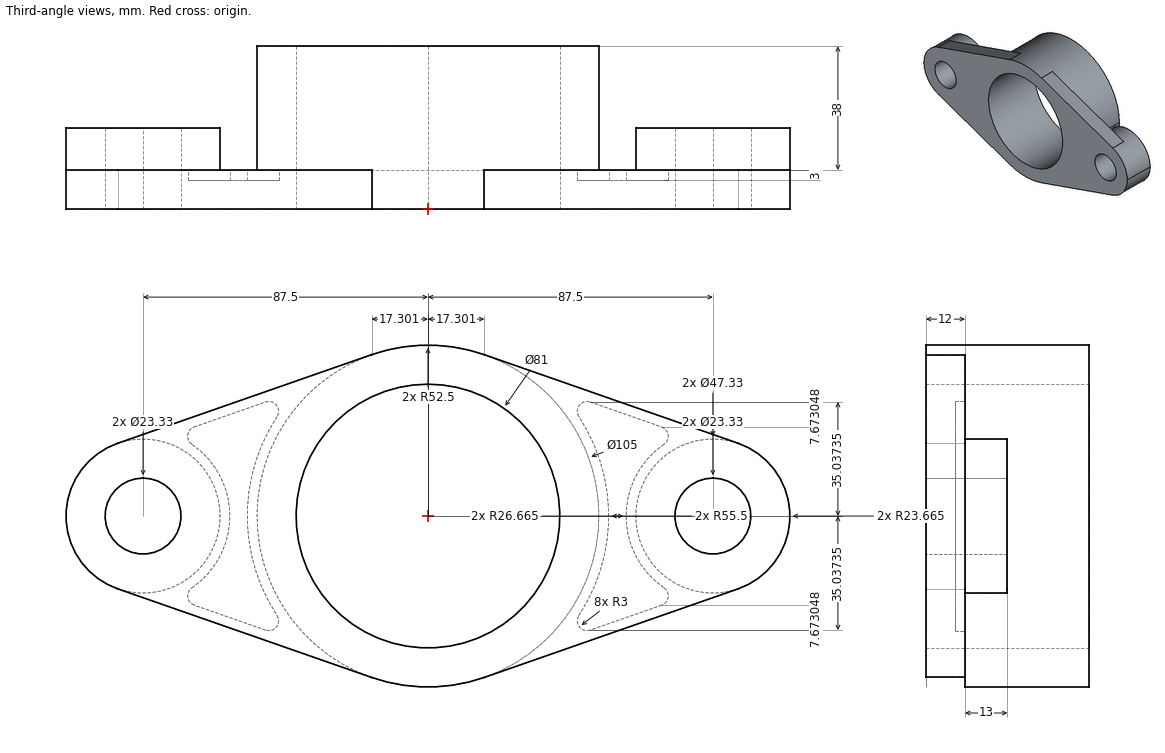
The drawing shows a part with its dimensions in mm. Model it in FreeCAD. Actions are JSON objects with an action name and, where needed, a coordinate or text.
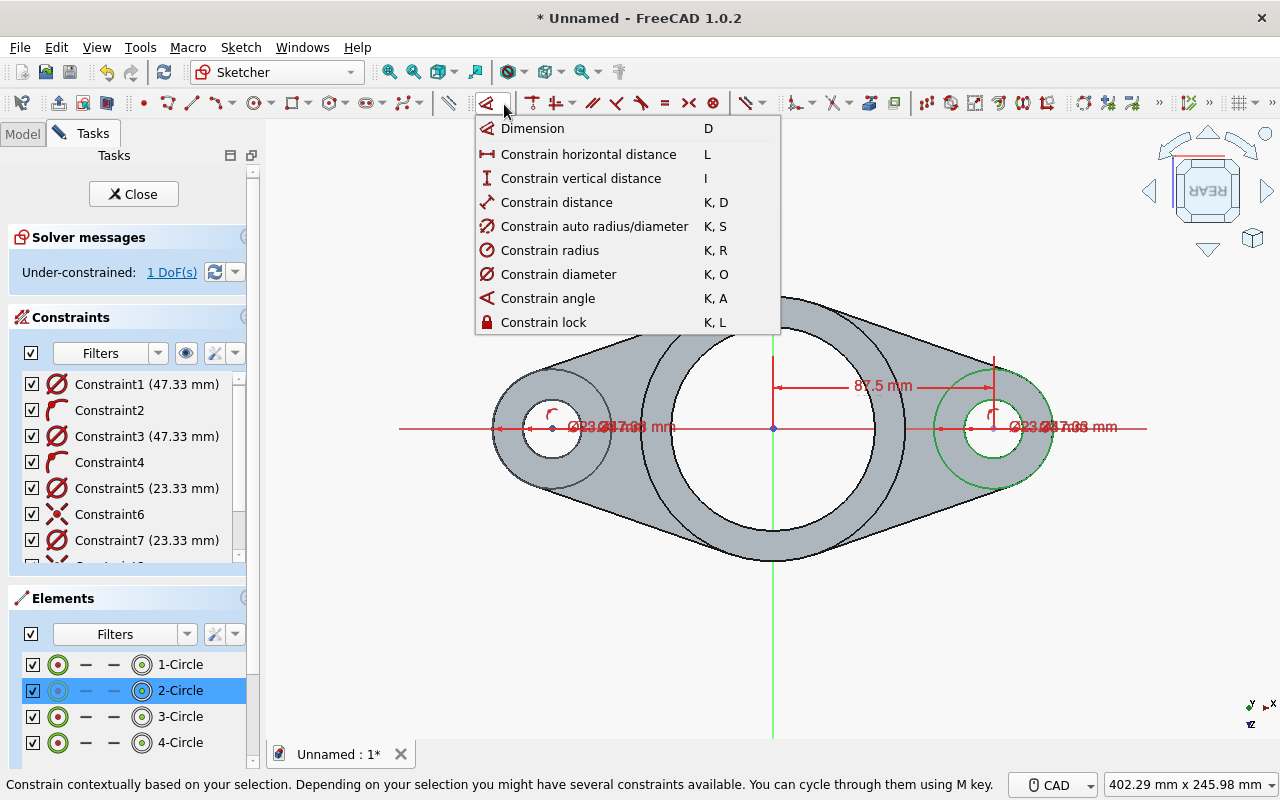
{"action": "left_click", "coordinate": [628, 154]}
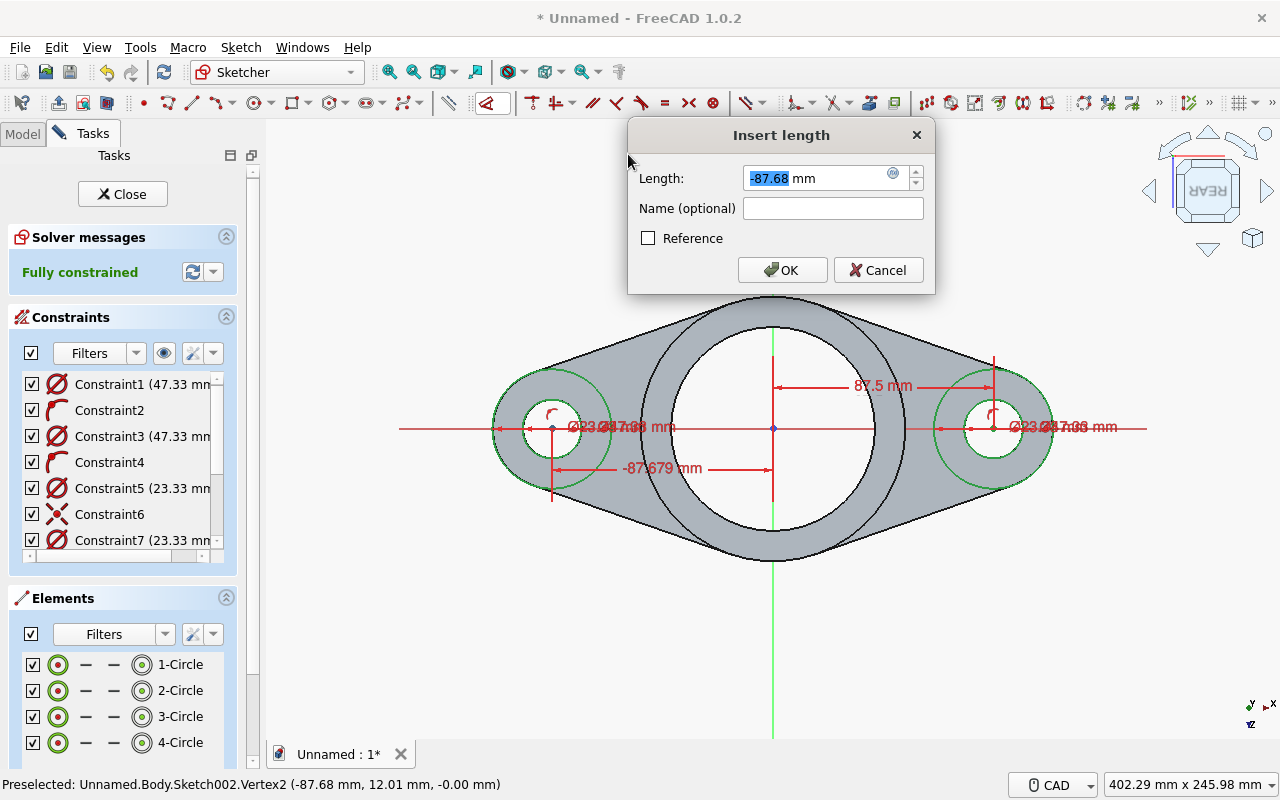
{"action": "type", "text": "-87.5"}
{"action": "key", "text": "Return"}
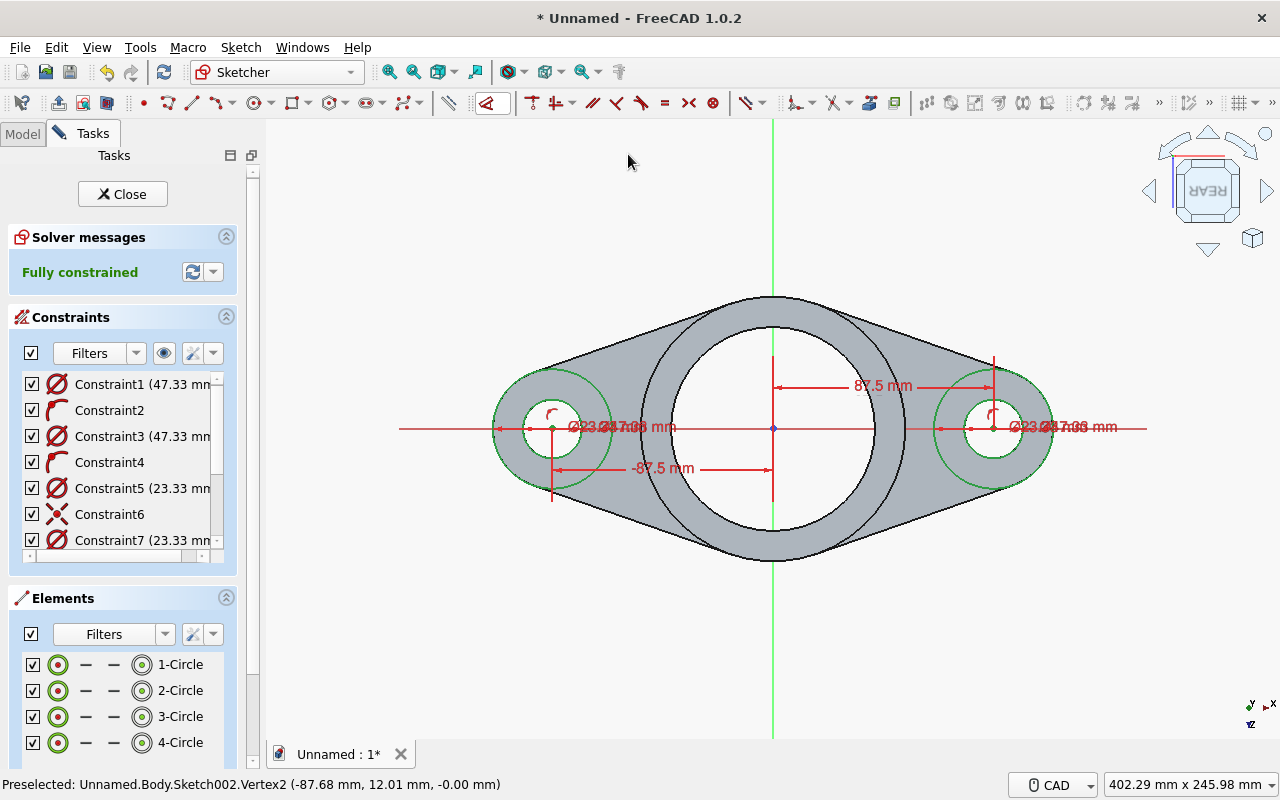
{"action": "left_click", "coordinate": [123, 194]}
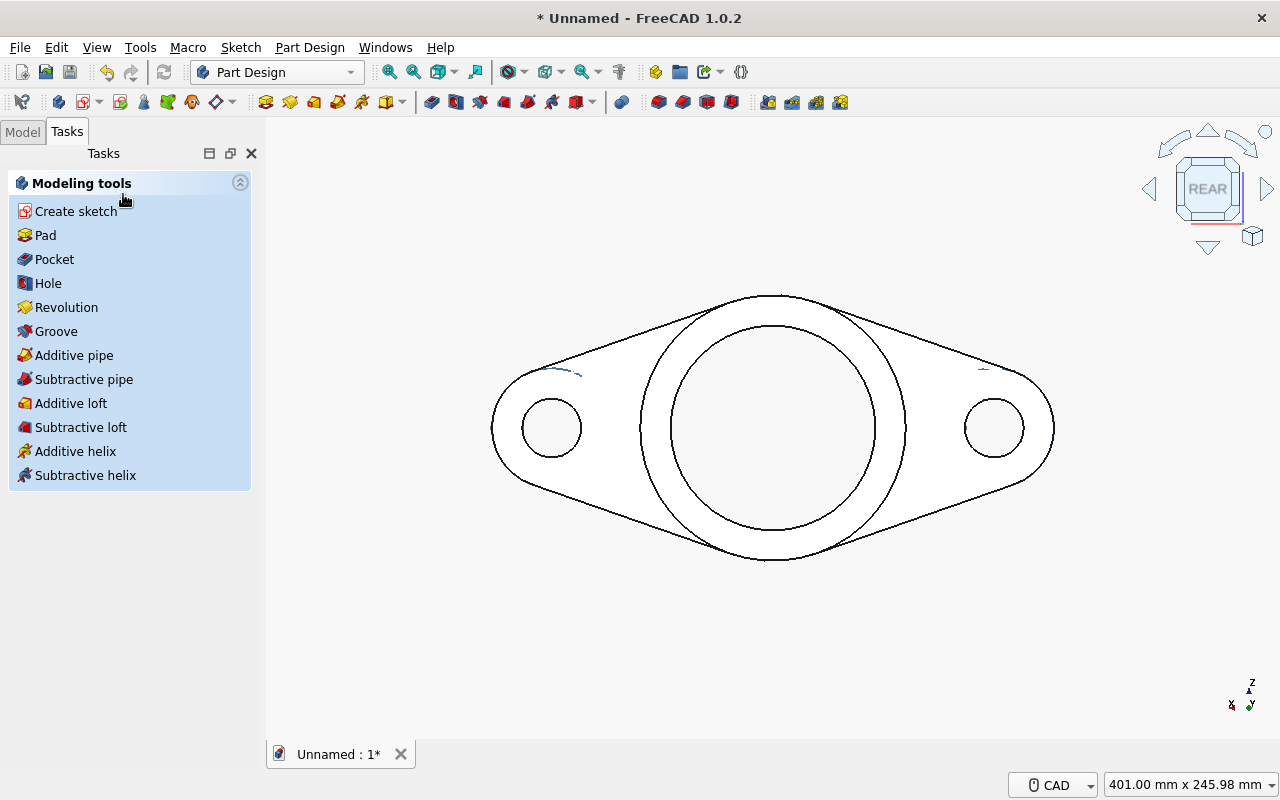
{"action": "left_click", "coordinate": [266, 102]}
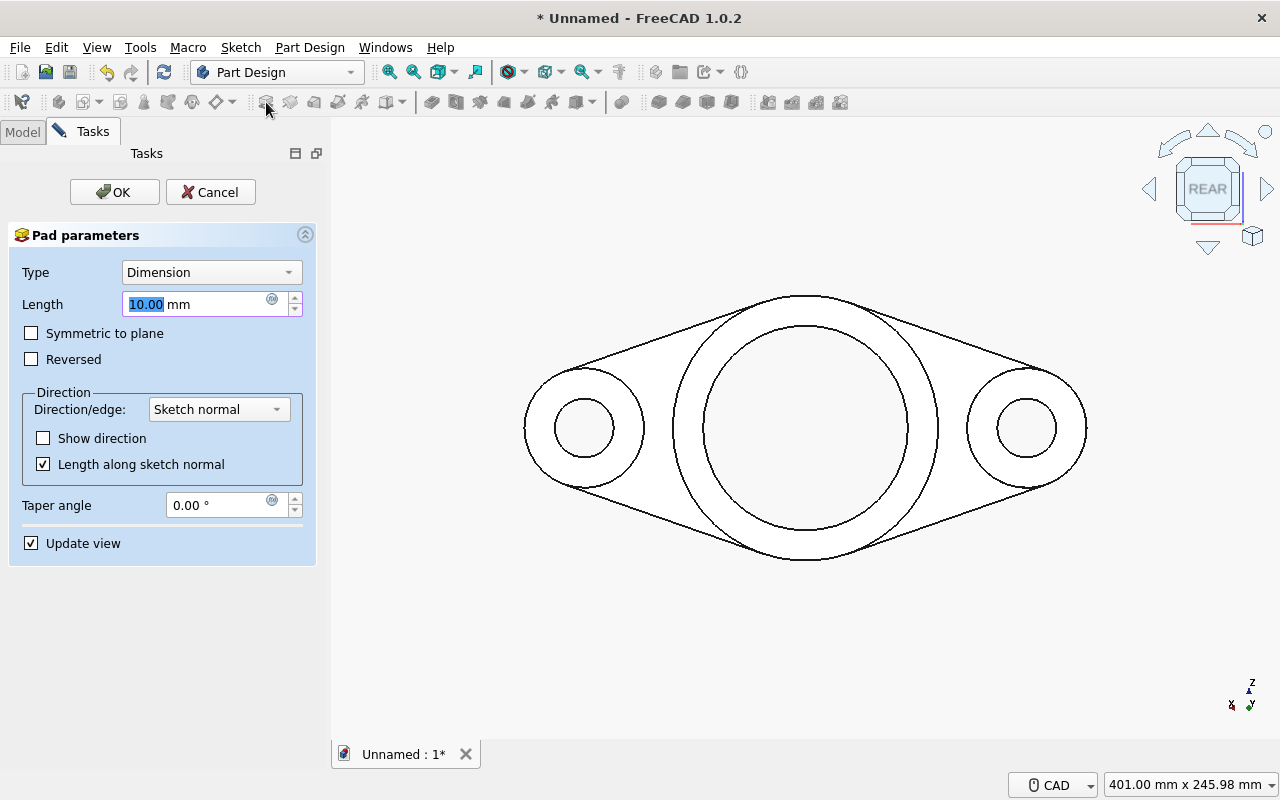
{"action": "type", "text": "13"}
{"action": "key", "text": "Tab"}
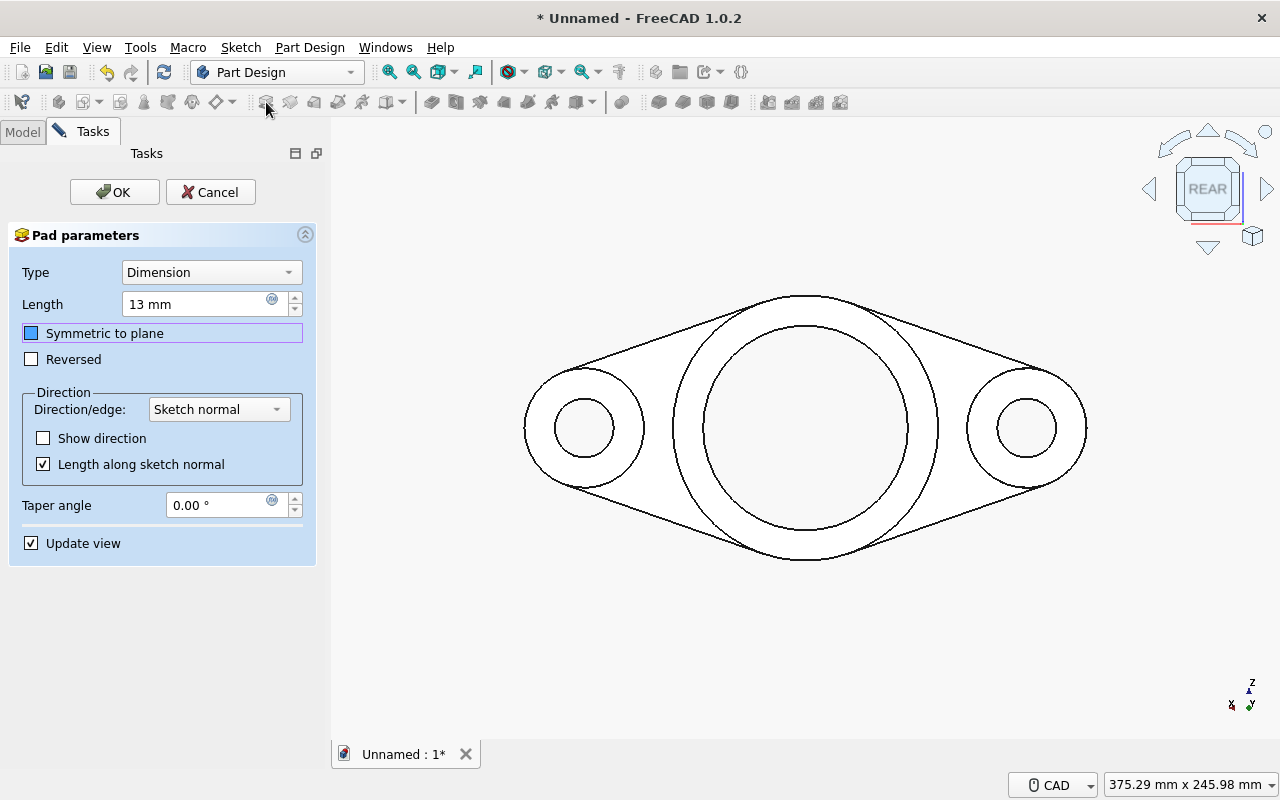
{"action": "left_click", "coordinate": [115, 192]}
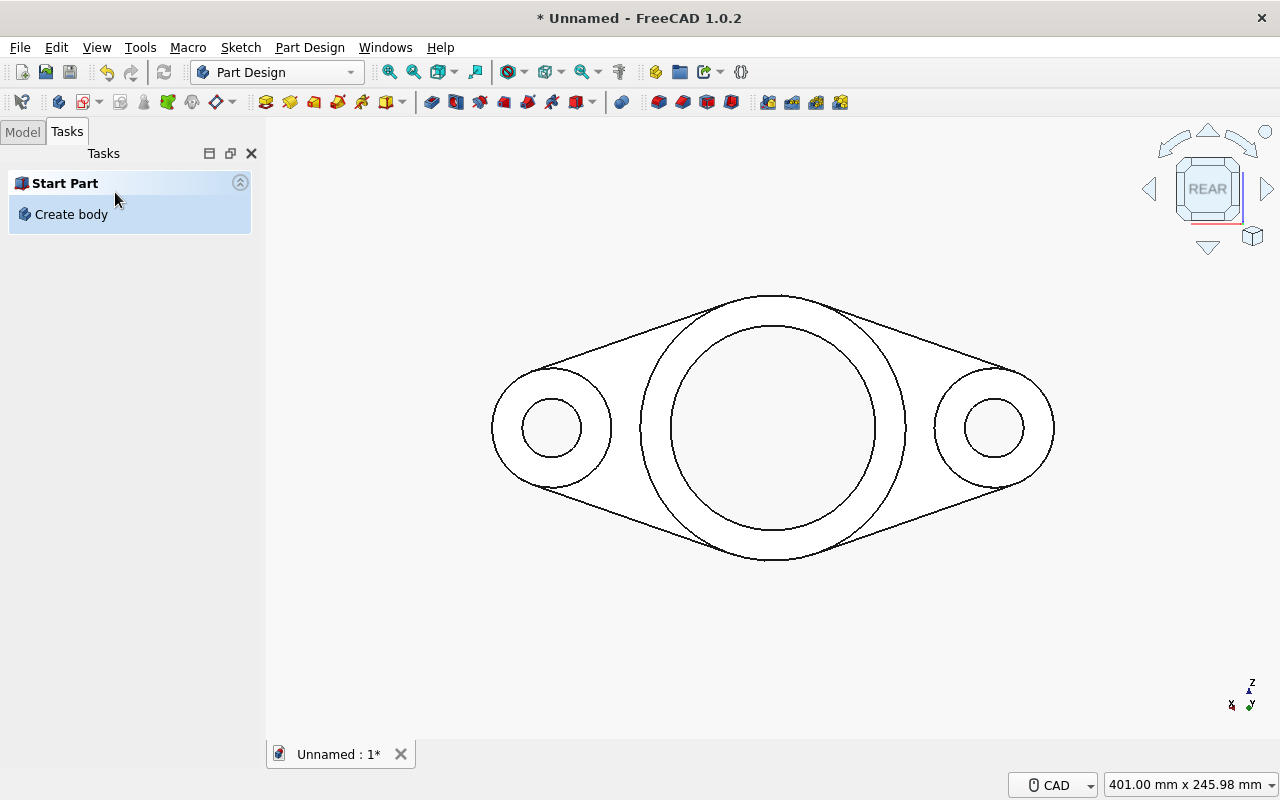
{"action": "left_click", "coordinate": [915, 355]}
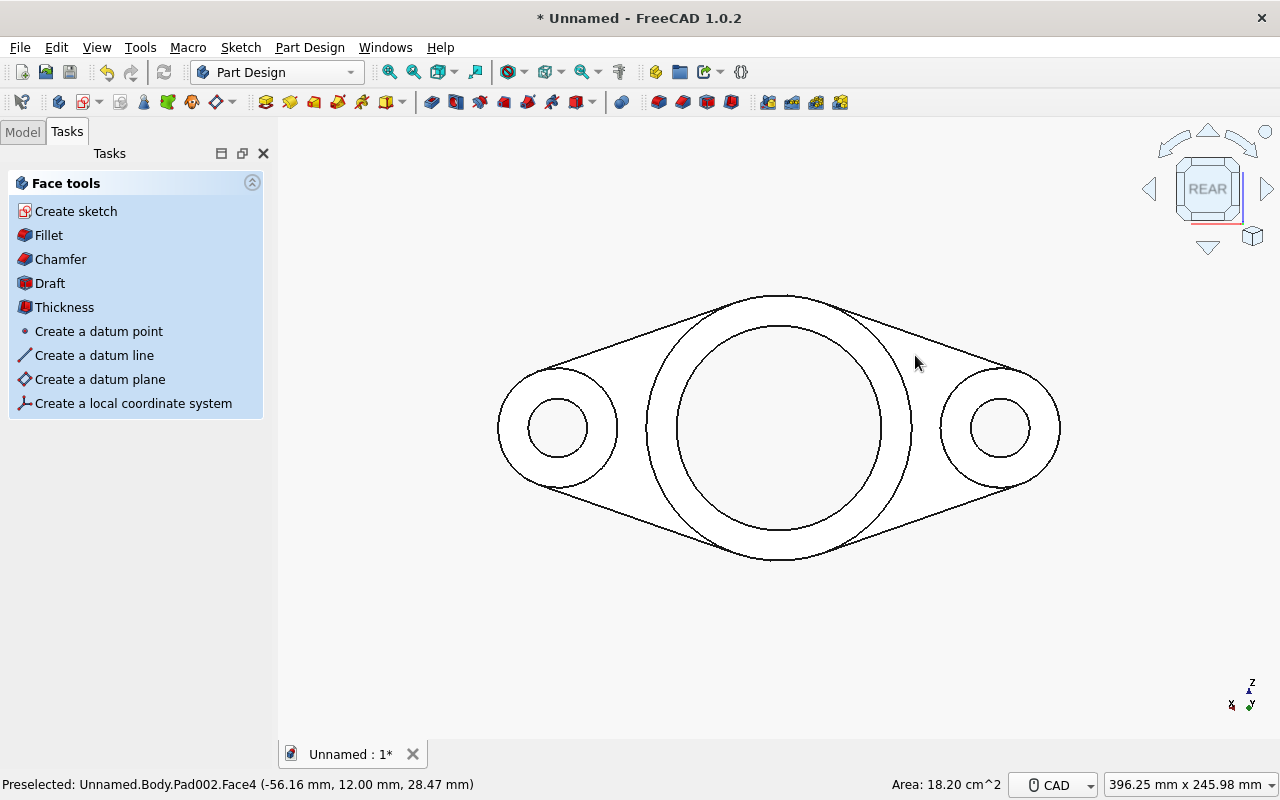
{"action": "left_click", "coordinate": [84, 102]}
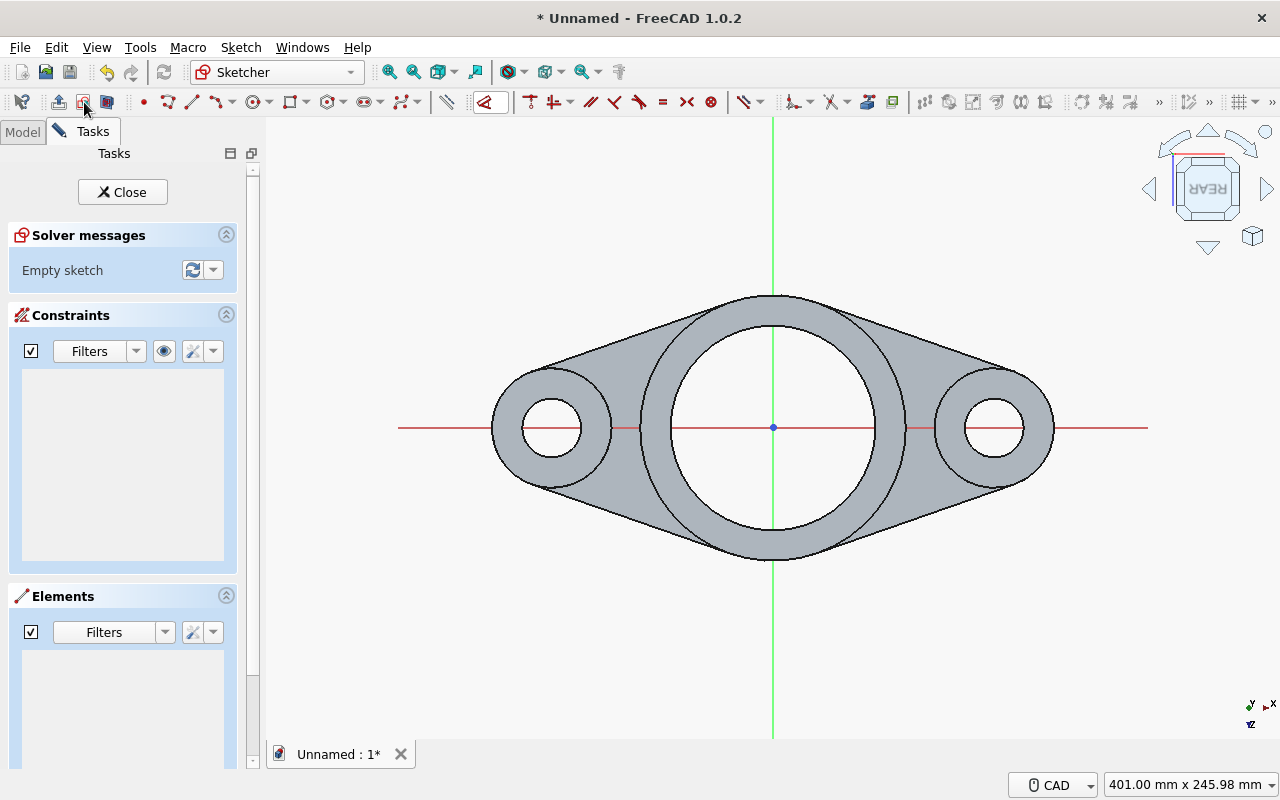
{"action": "left_click", "coordinate": [108, 102]}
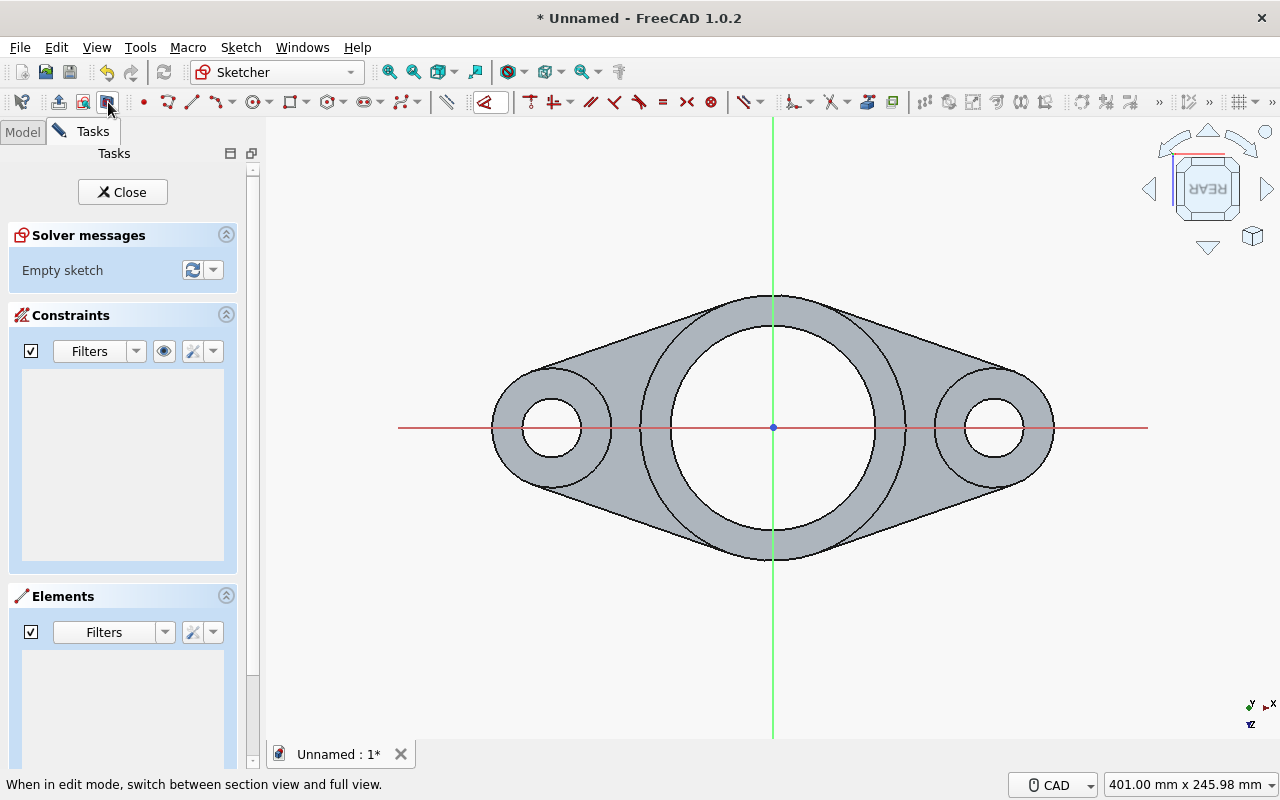
{"action": "scroll", "coordinate": [912, 428], "scroll_direction": "up", "scroll_amount": 2}